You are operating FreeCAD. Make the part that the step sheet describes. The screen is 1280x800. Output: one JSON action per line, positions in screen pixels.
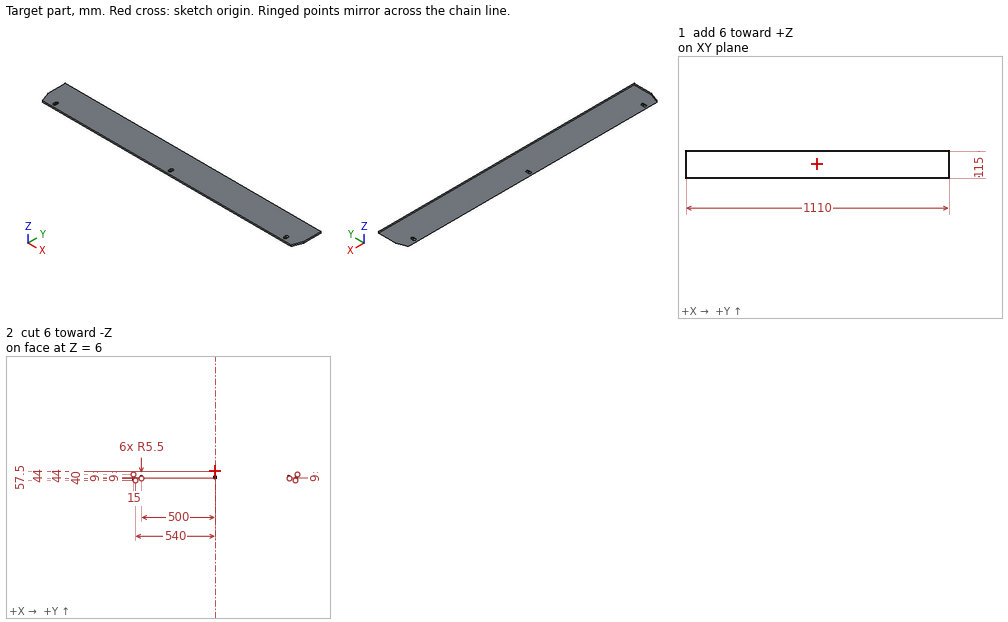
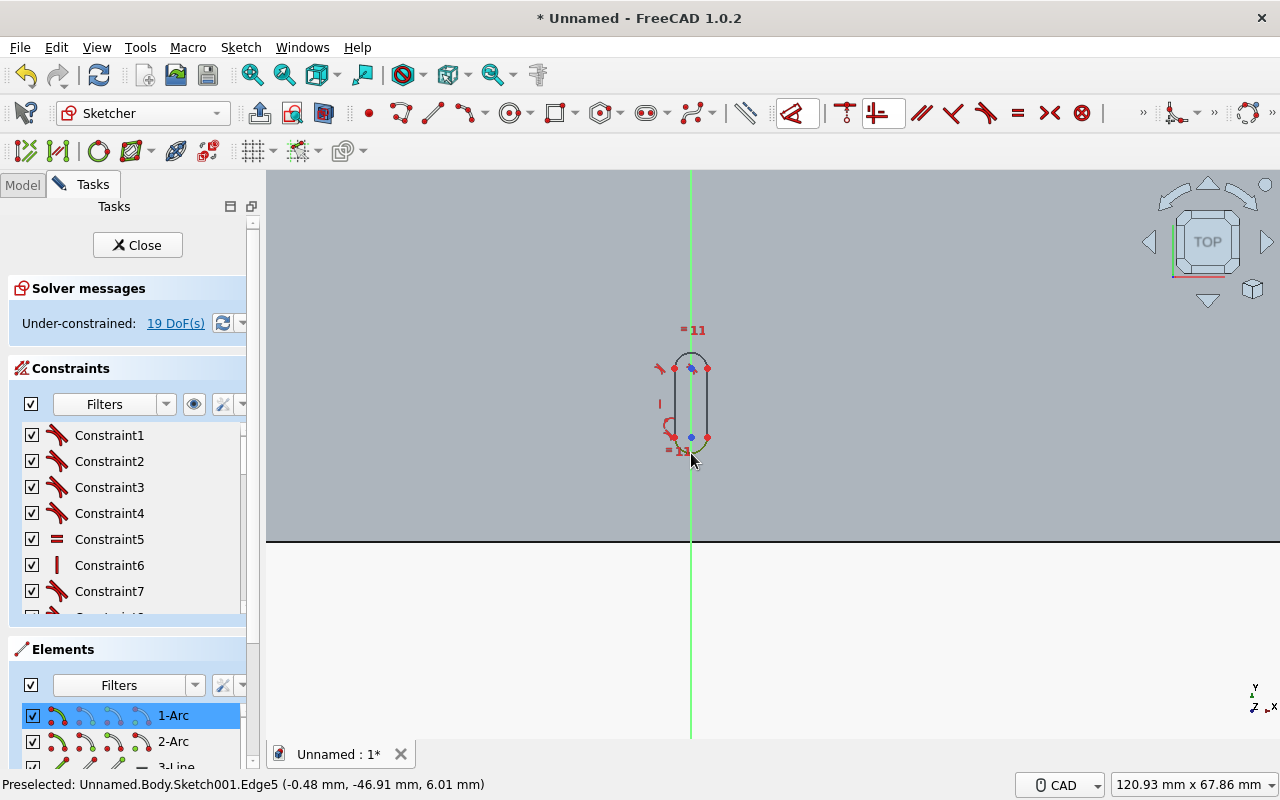
{"action": "scroll", "coordinate": [705, 464], "scroll_direction": "down", "scroll_amount": 14}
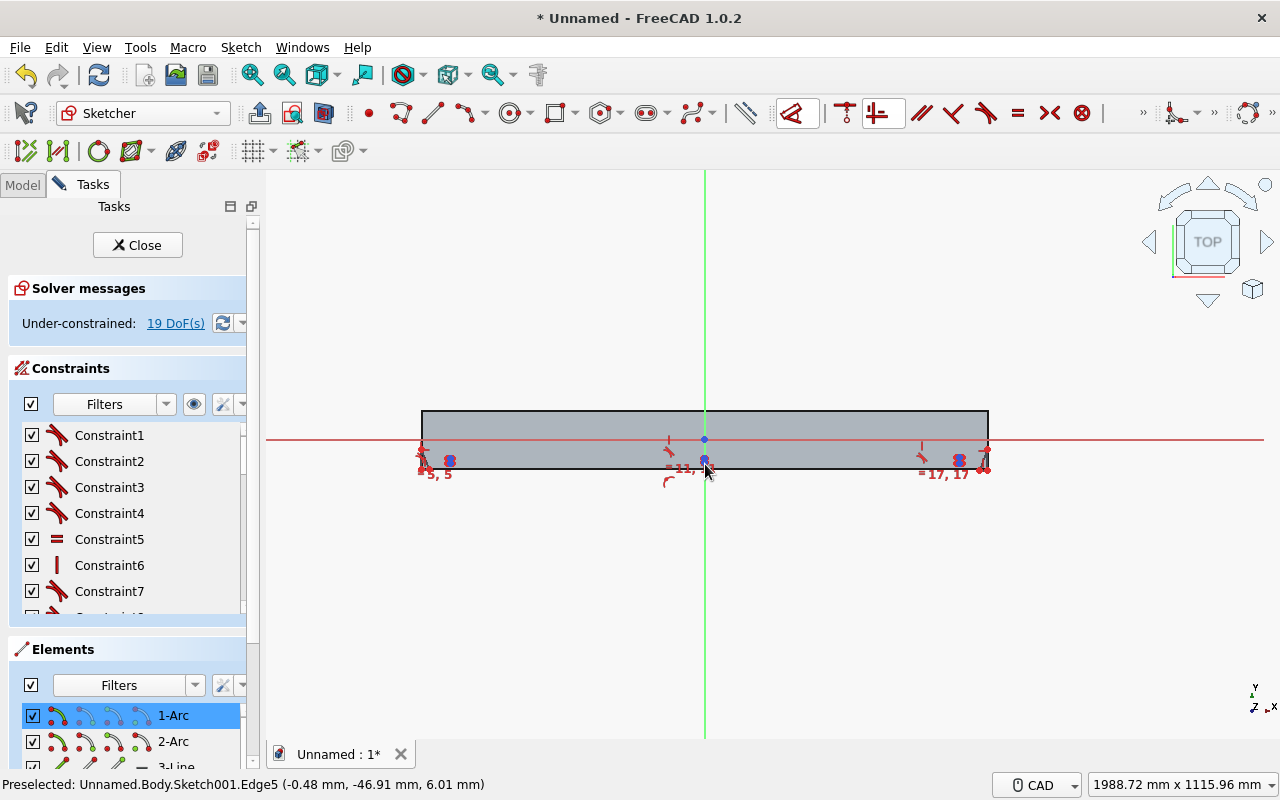
{"action": "scroll", "coordinate": [958, 466], "scroll_direction": "up", "scroll_amount": 8}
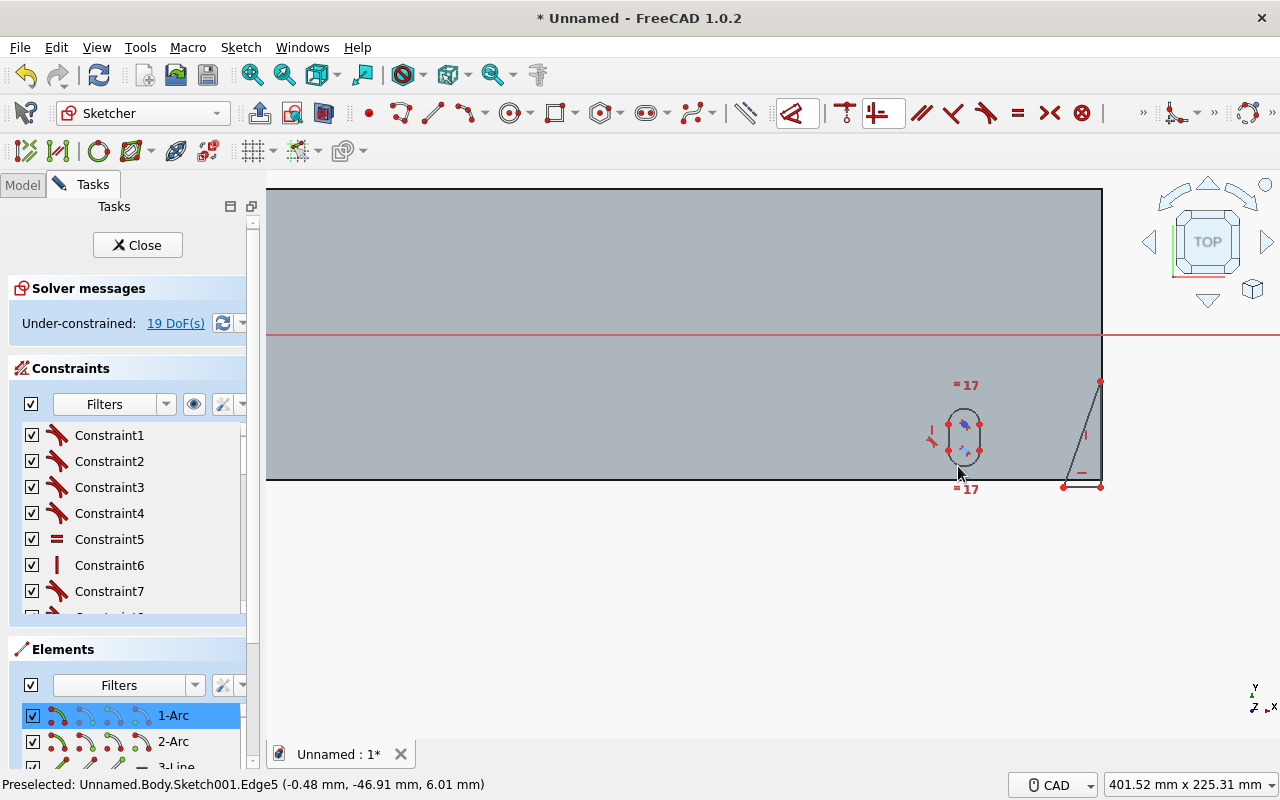
{"action": "left_click", "coordinate": [955, 463]}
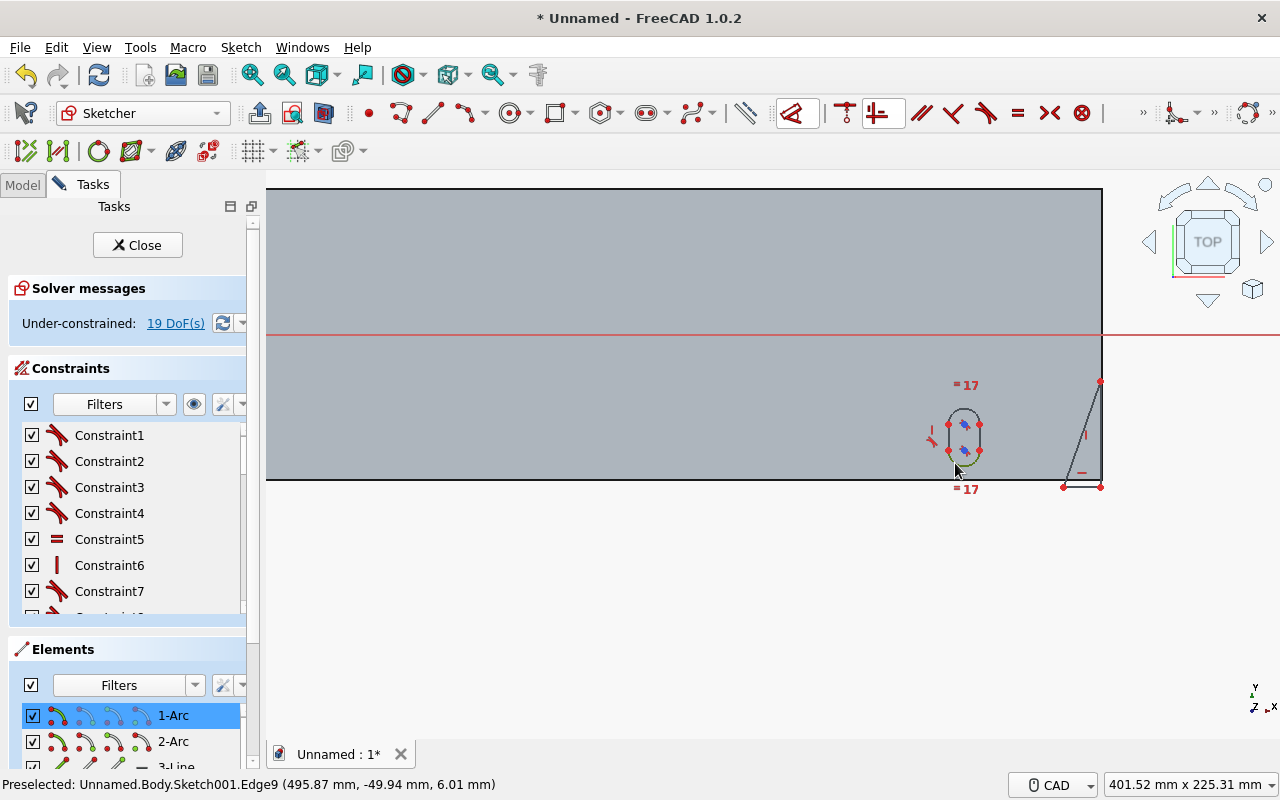
{"action": "left_click", "coordinate": [1018, 114]}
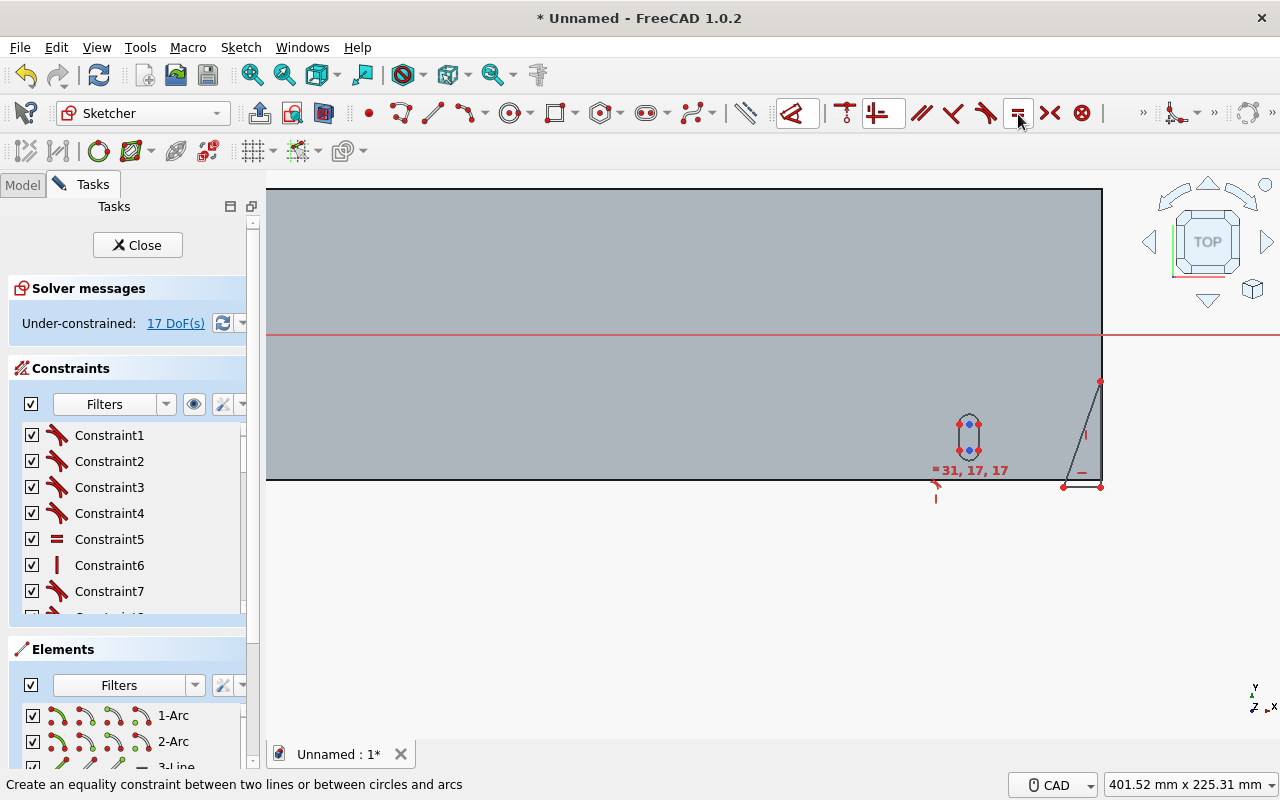
{"action": "scroll", "coordinate": [959, 466], "scroll_direction": "down", "scroll_amount": 8}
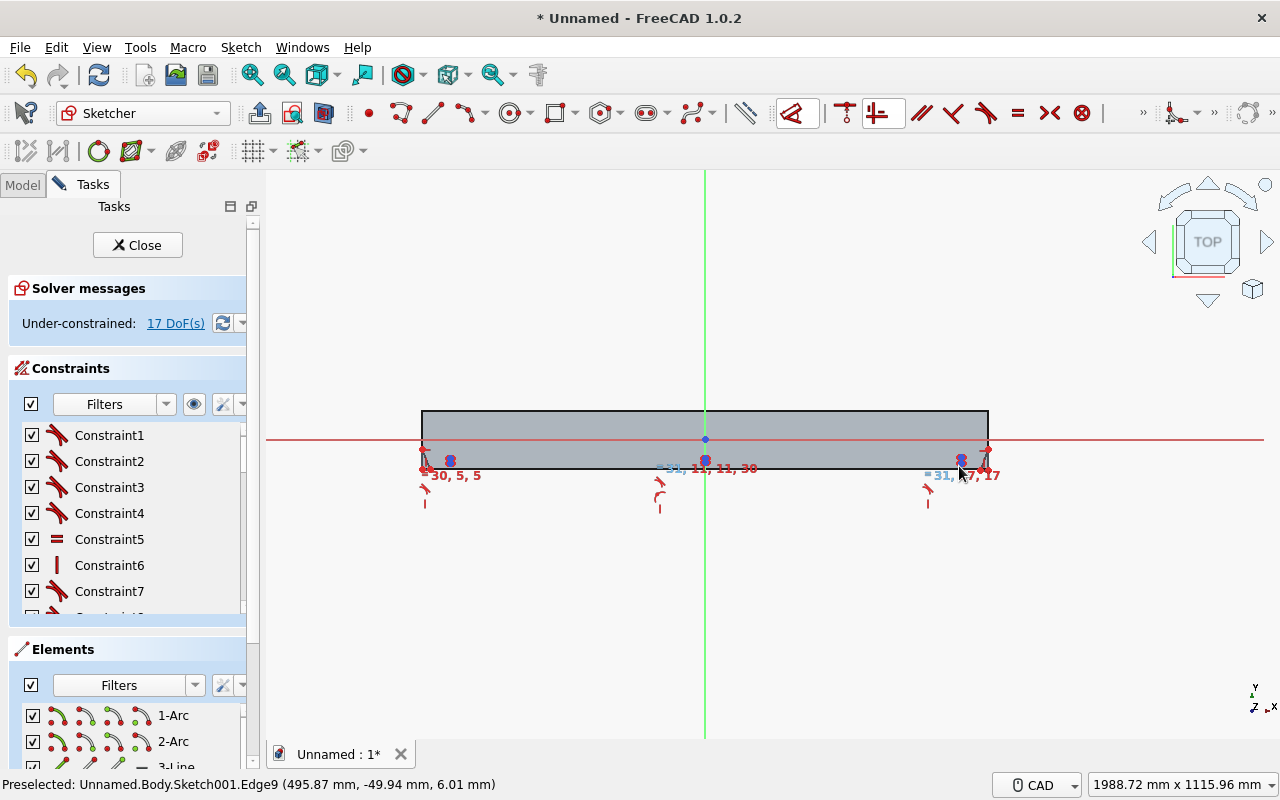
{"action": "scroll", "coordinate": [451, 464], "scroll_direction": "up", "scroll_amount": 10}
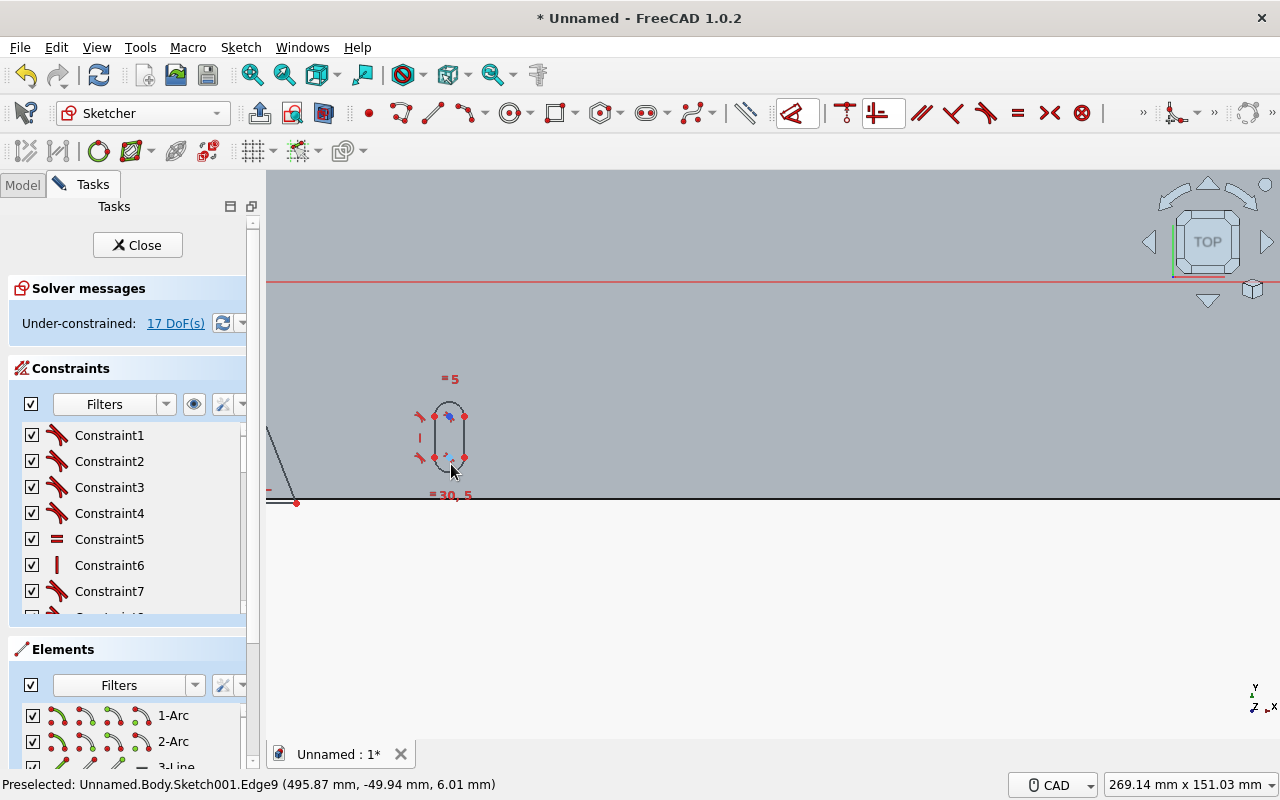
{"action": "left_click", "coordinate": [449, 458]}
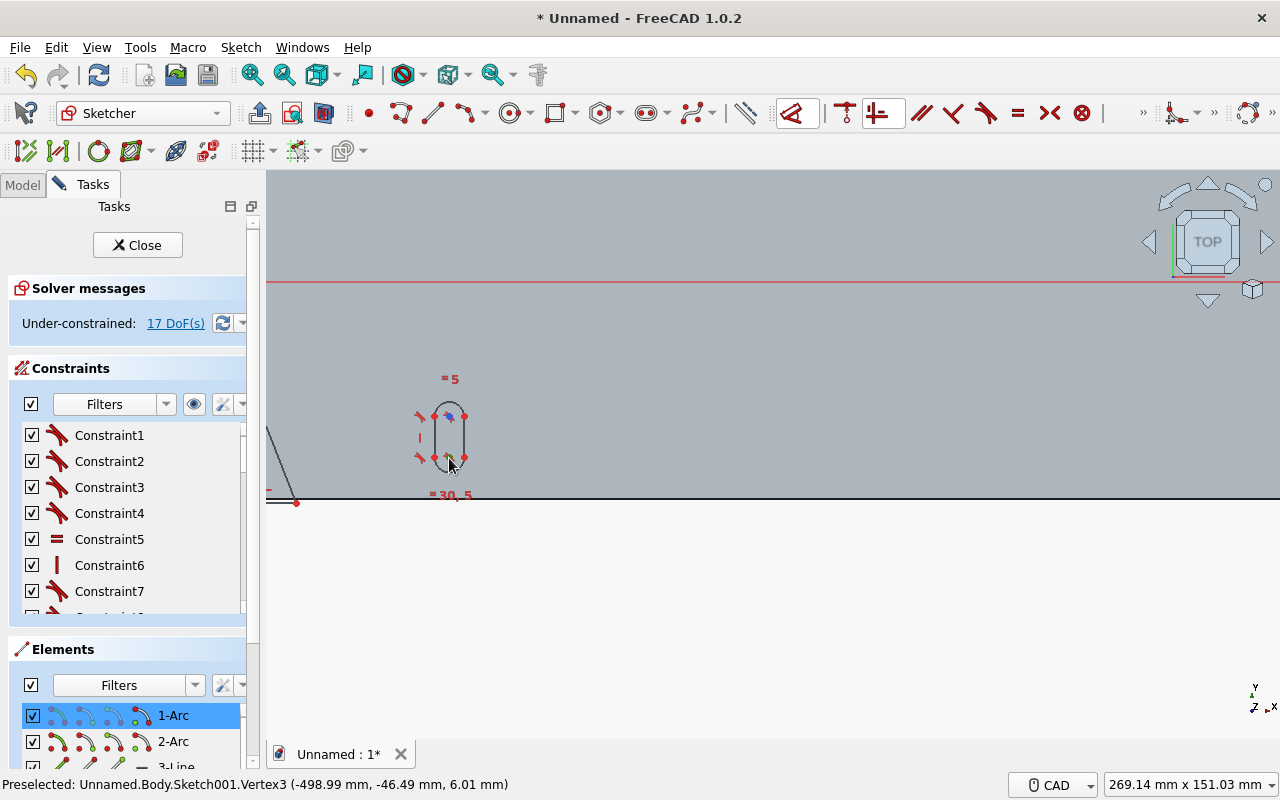
{"action": "scroll", "coordinate": [450, 464], "scroll_direction": "down", "scroll_amount": 10}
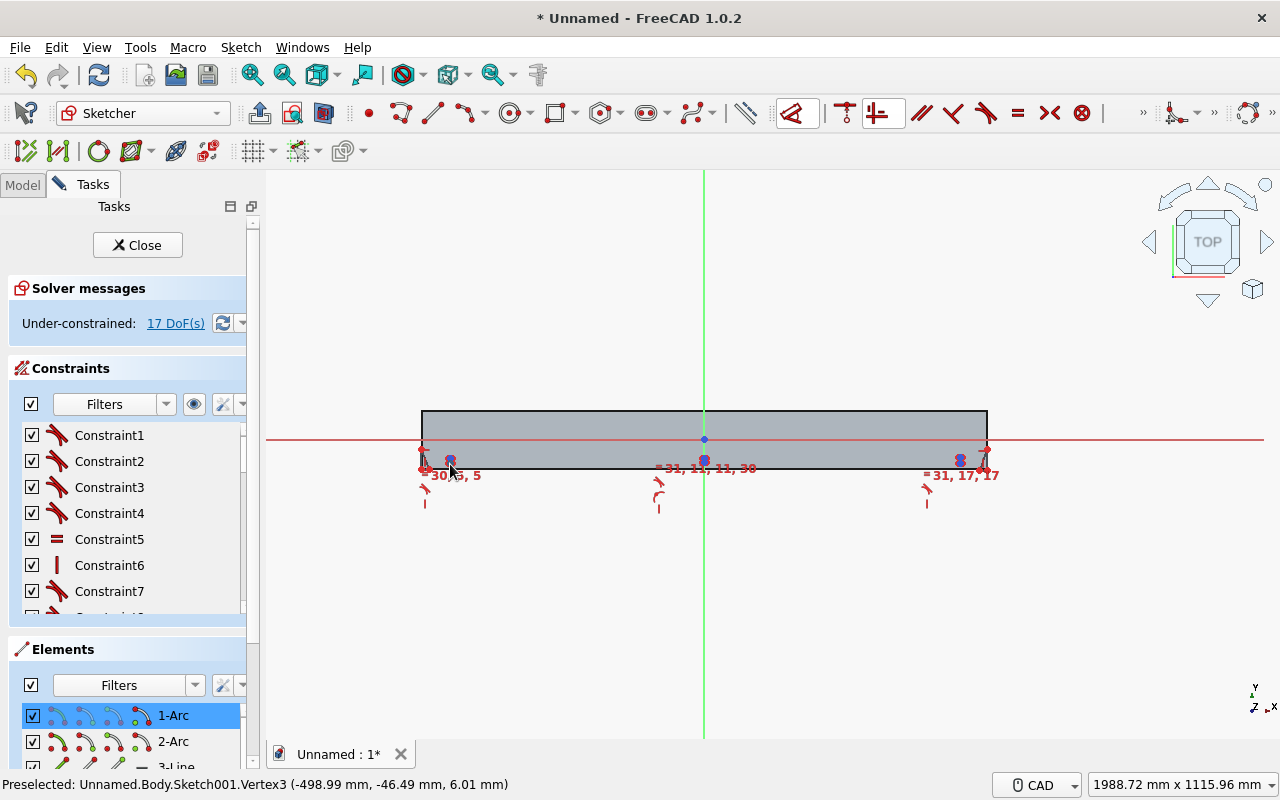
{"action": "scroll", "coordinate": [961, 463], "scroll_direction": "up", "scroll_amount": 10}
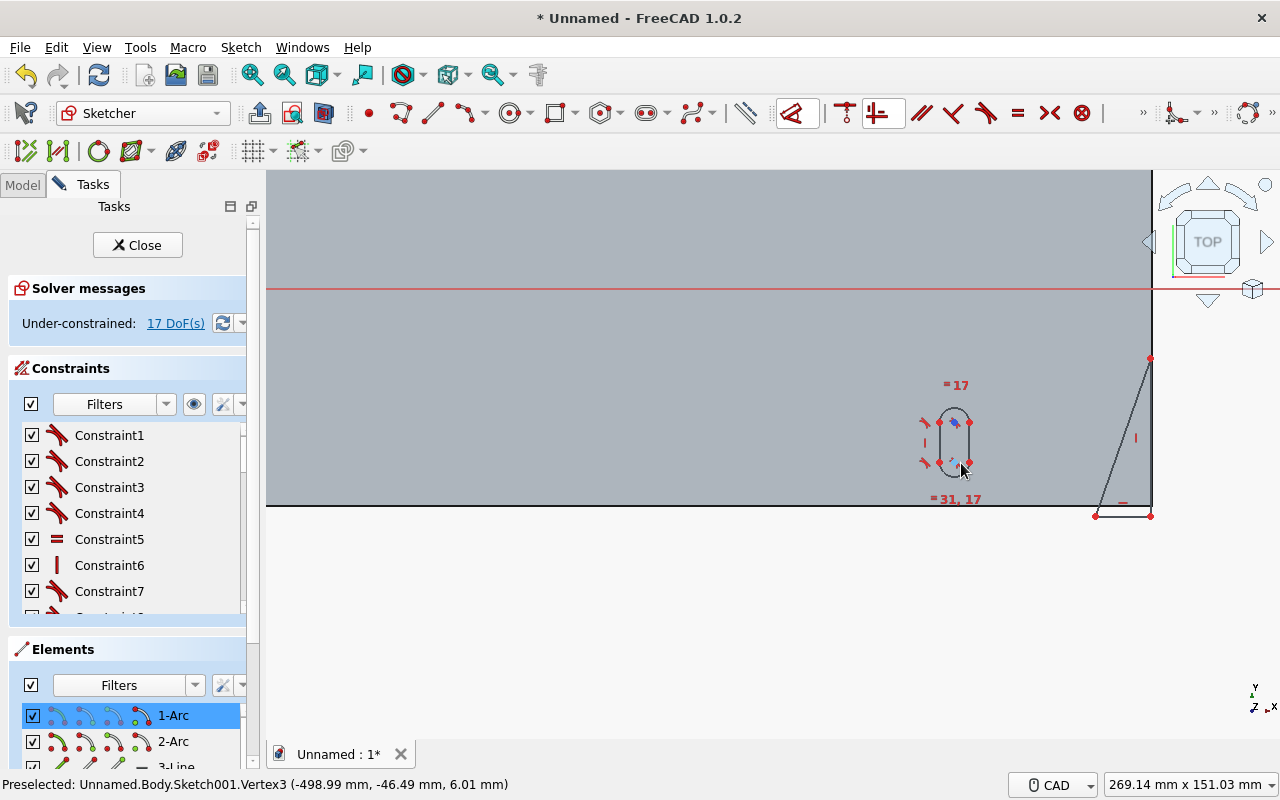
{"action": "left_click", "coordinate": [955, 462]}